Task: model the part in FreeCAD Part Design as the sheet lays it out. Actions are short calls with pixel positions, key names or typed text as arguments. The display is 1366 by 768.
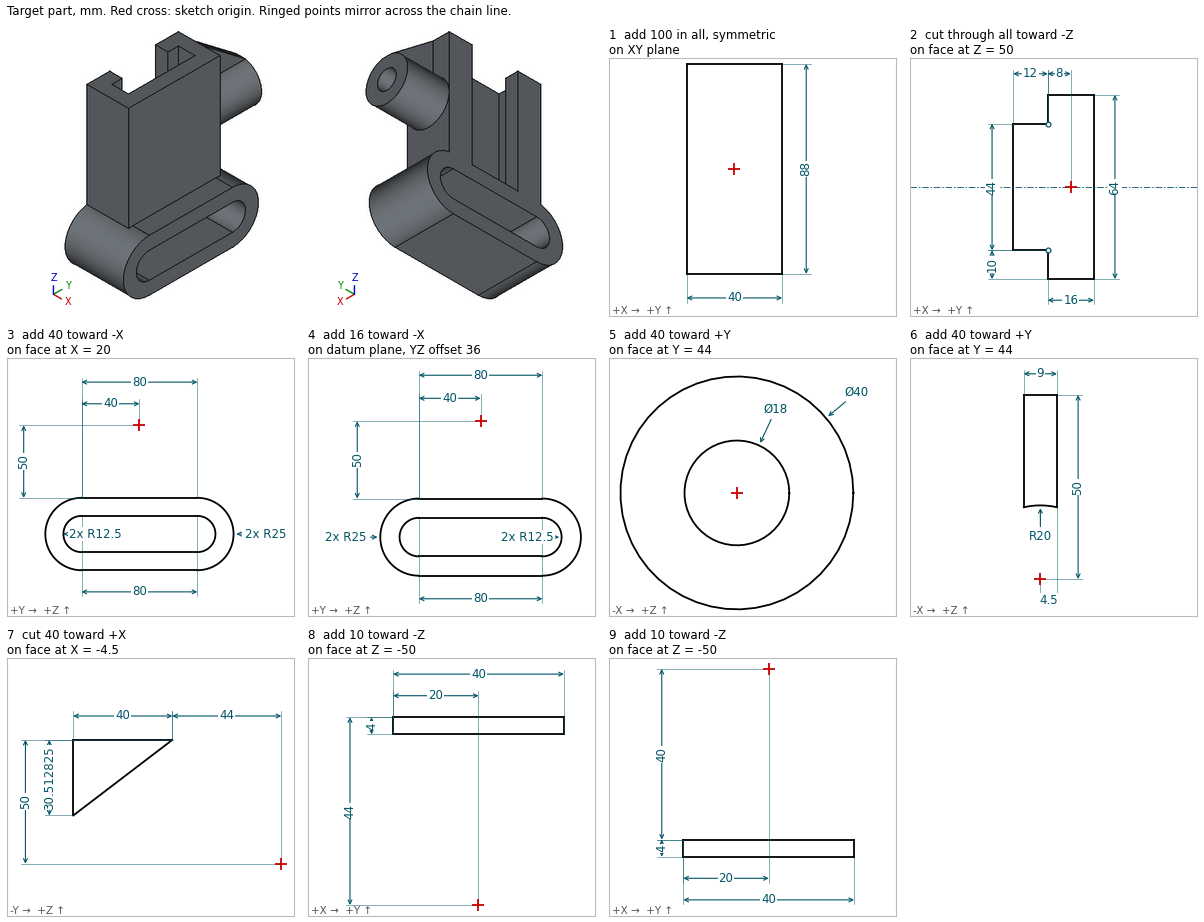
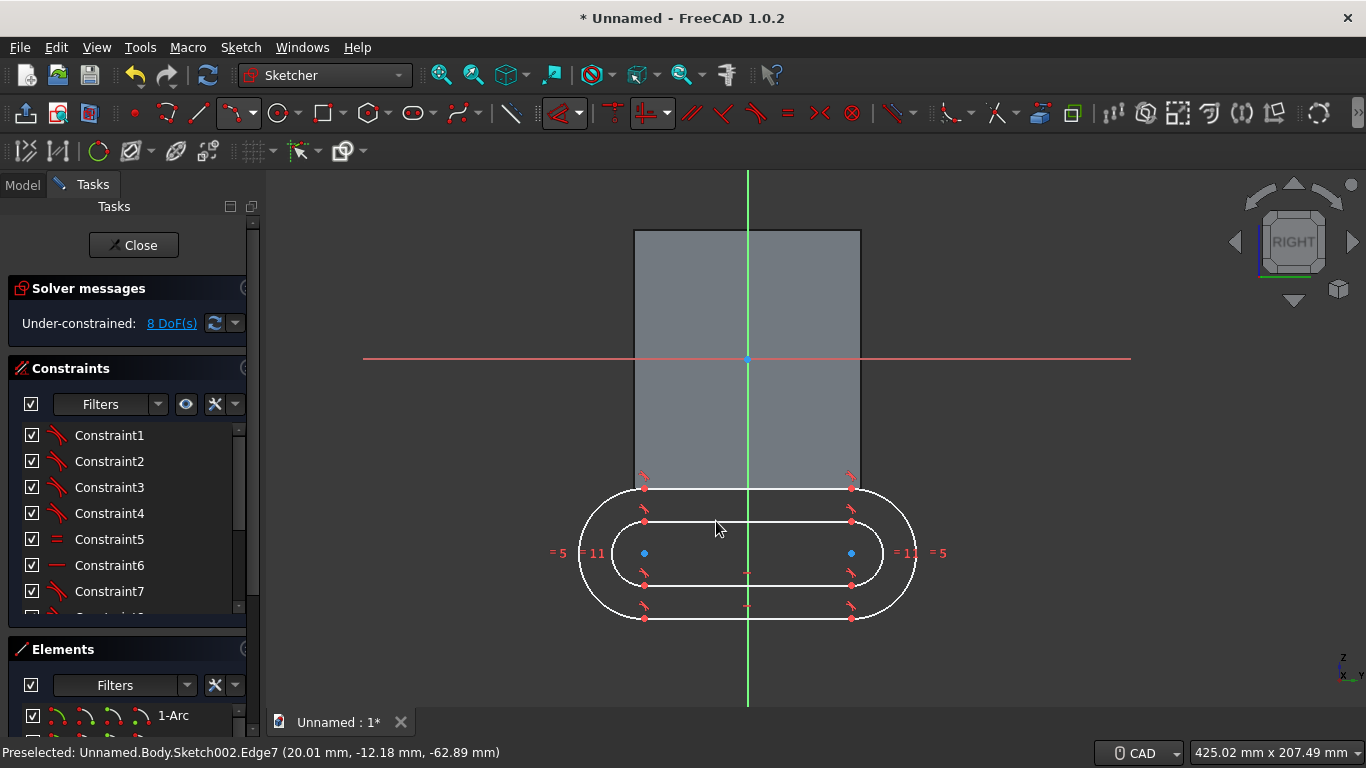
click(591, 516)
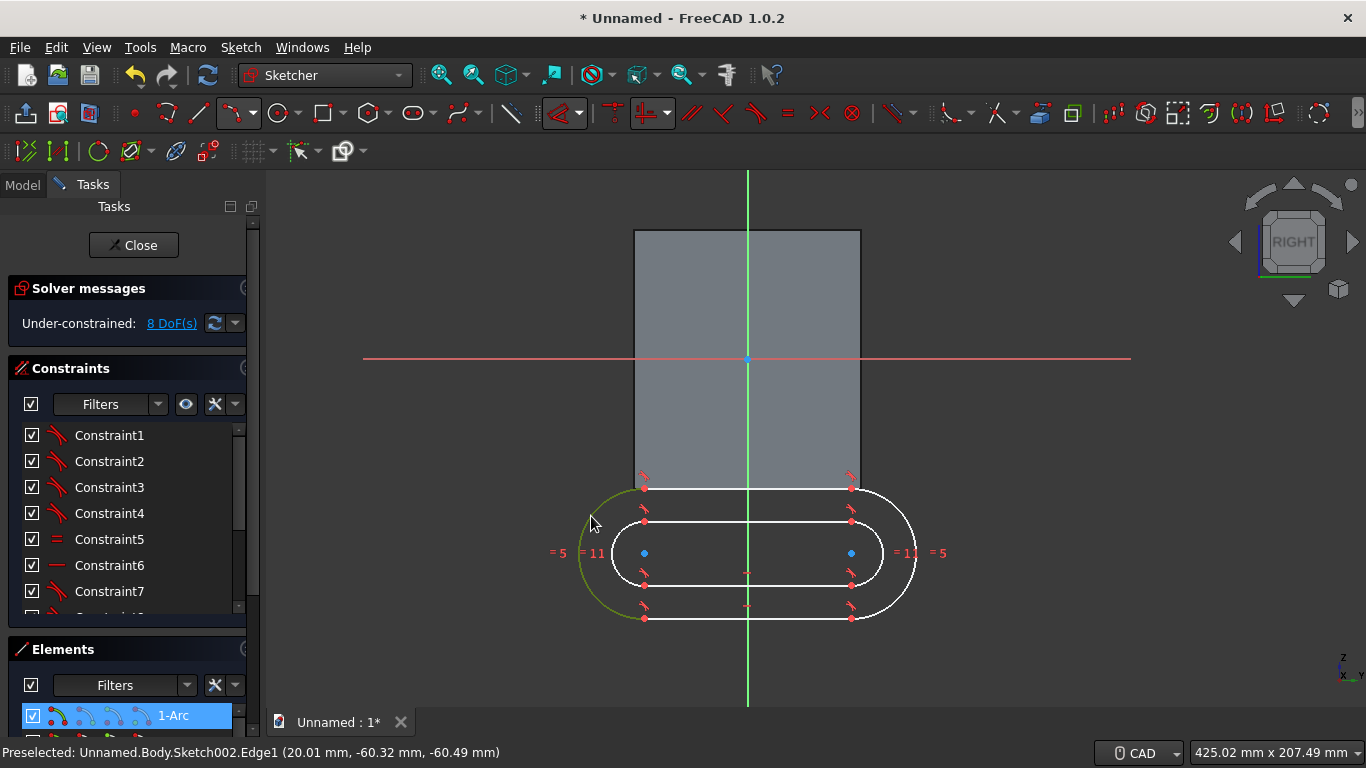
click(618, 535)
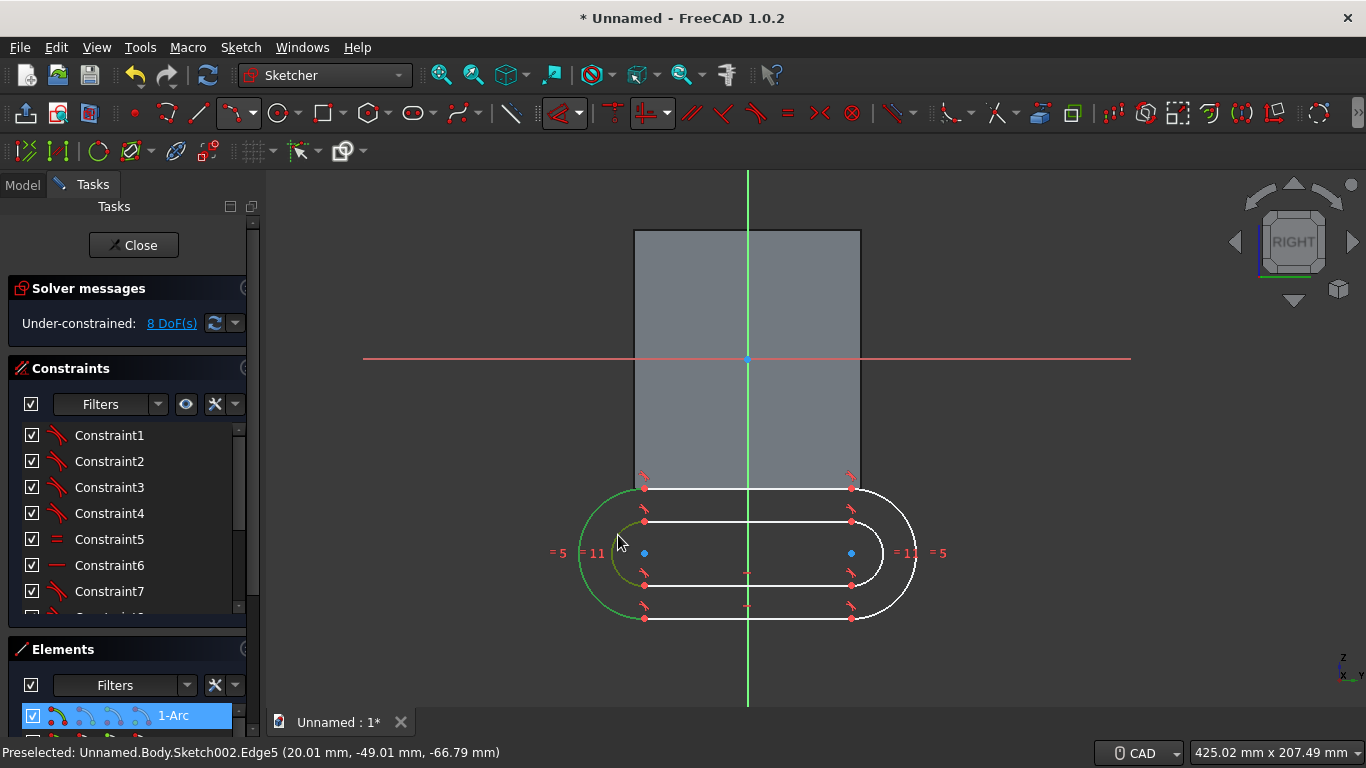
key(c)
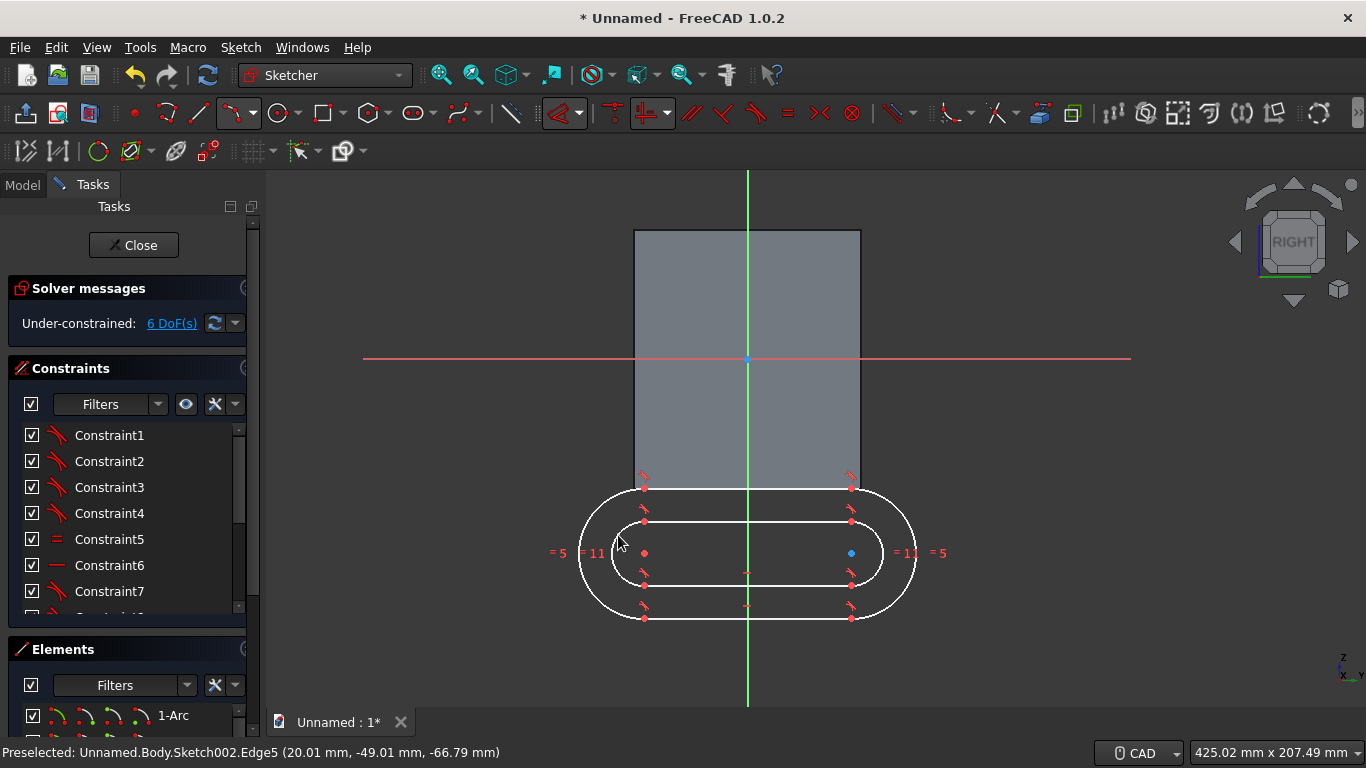
click(591, 516)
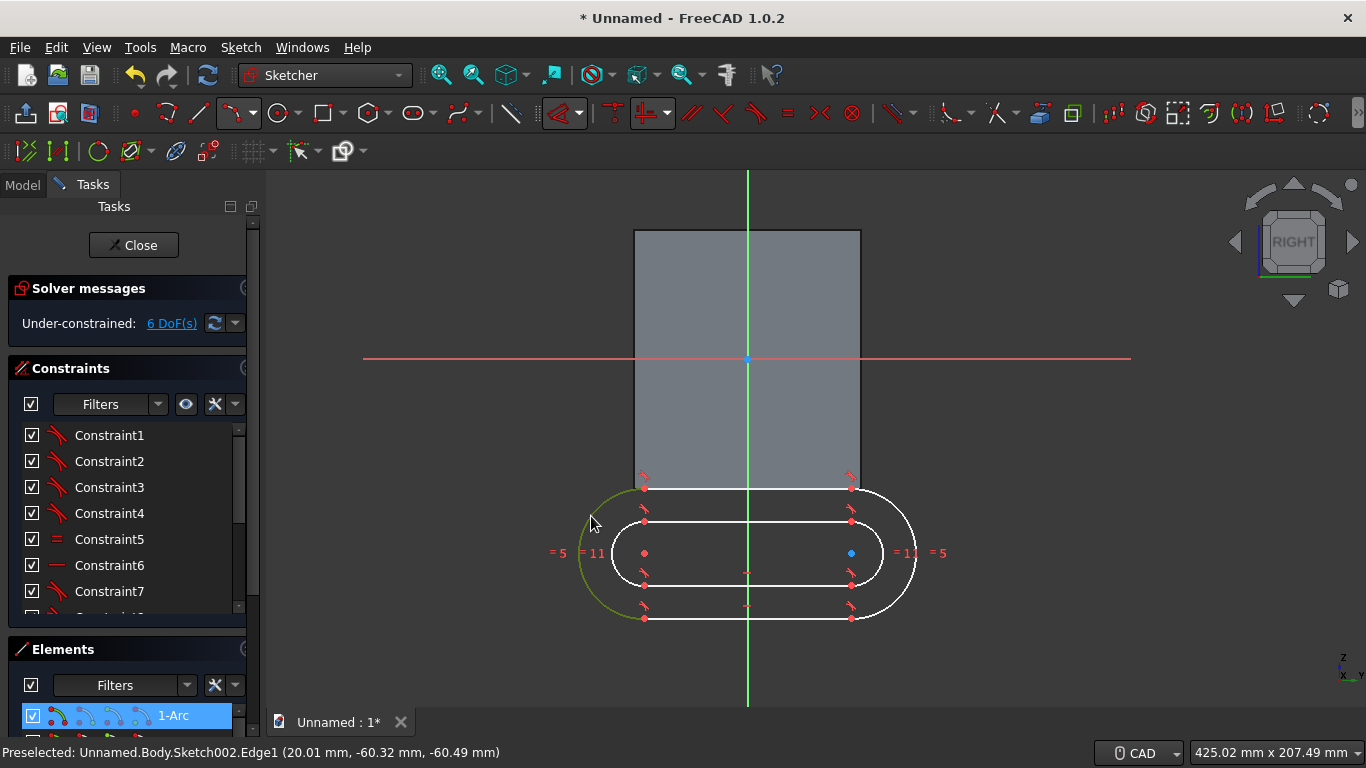
click(582, 114)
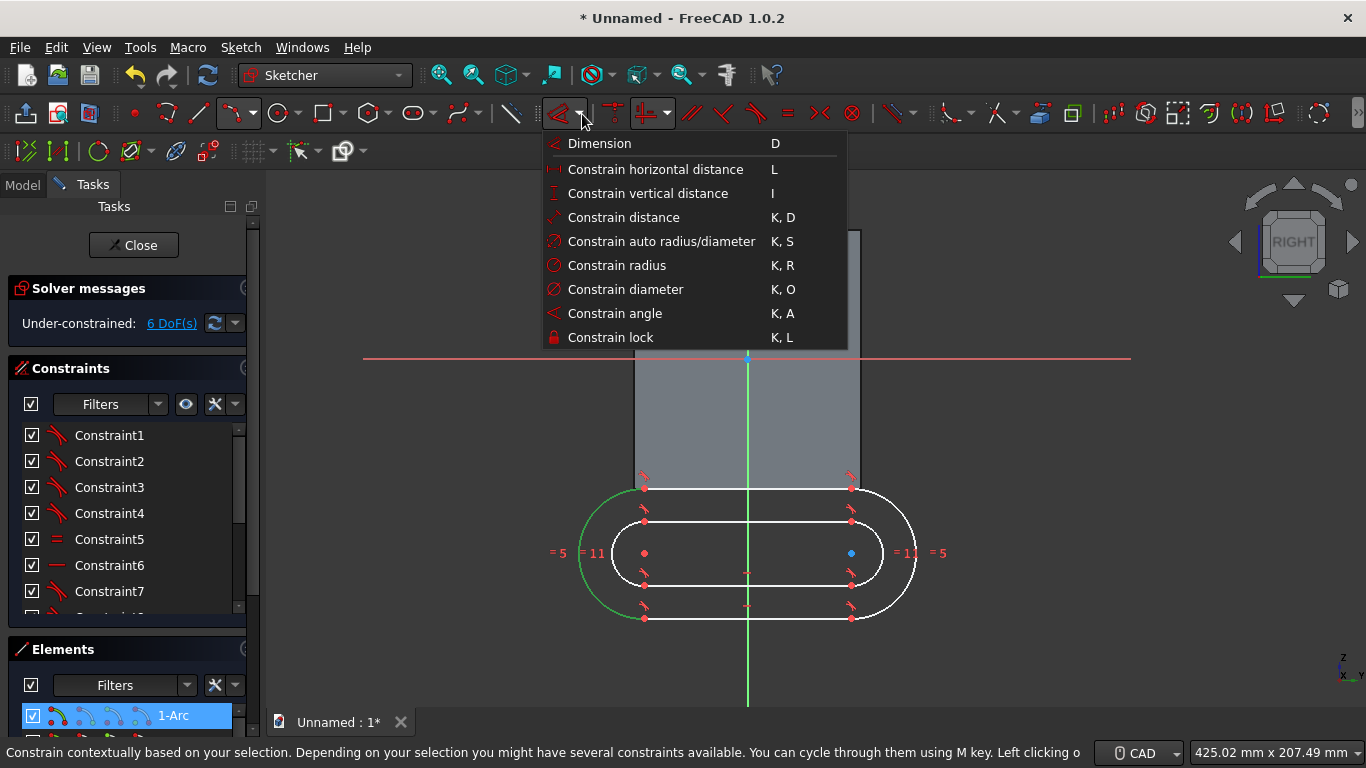
click(695, 265)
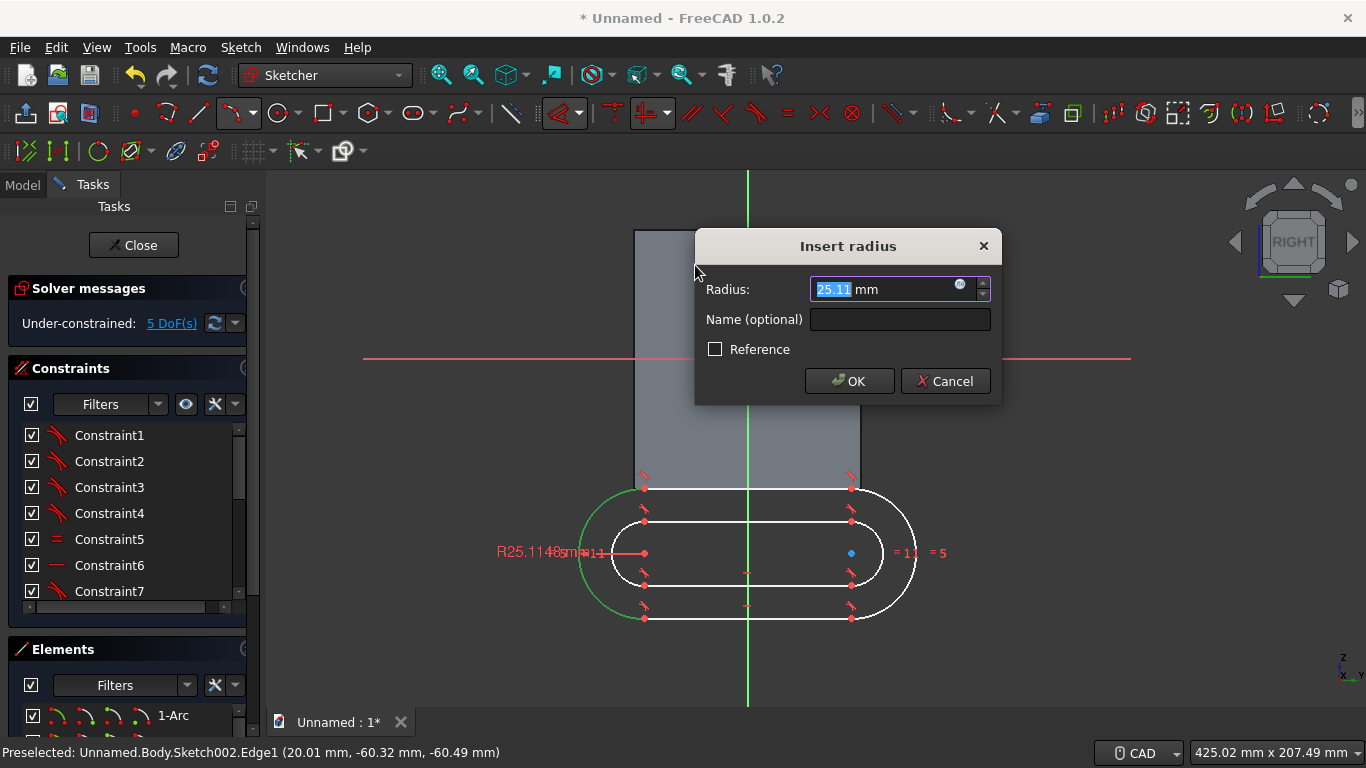
text(25)
key(Return)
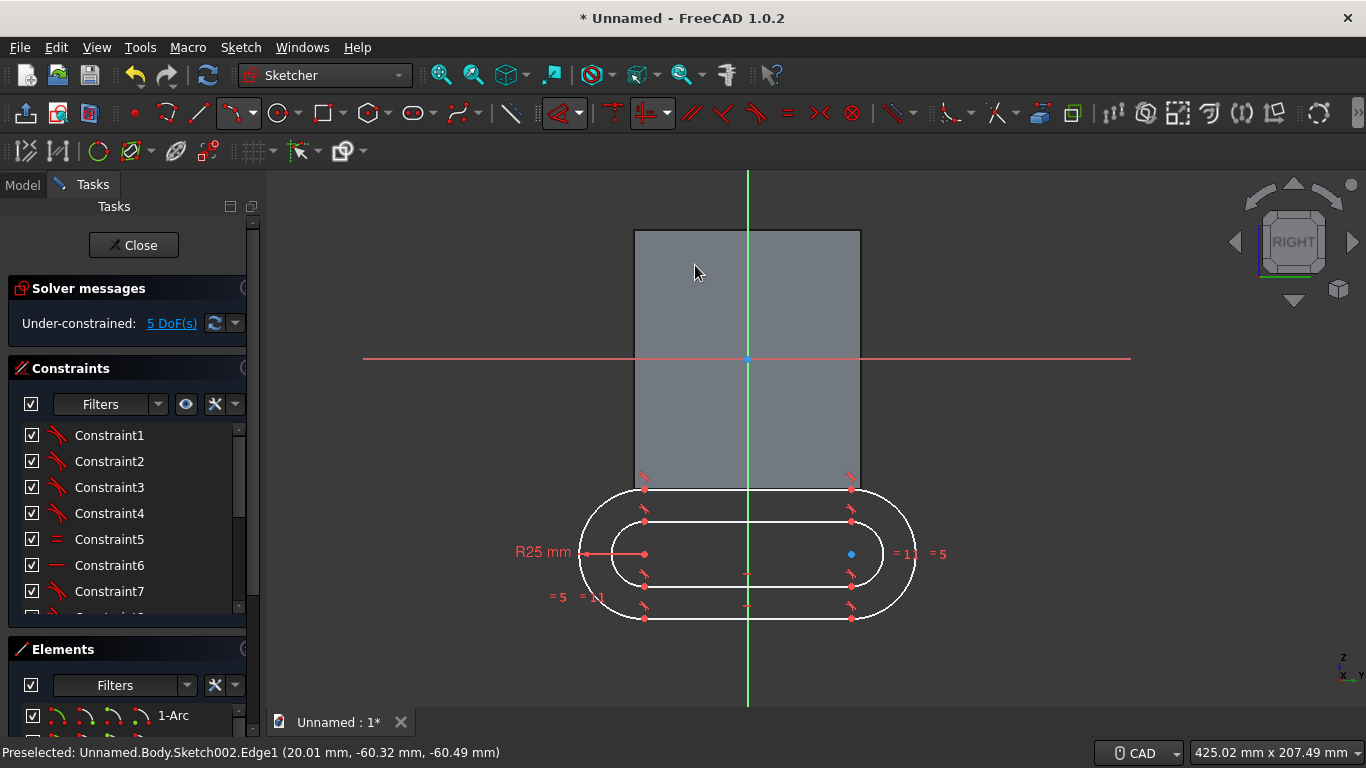
scroll(618, 535, up, 2)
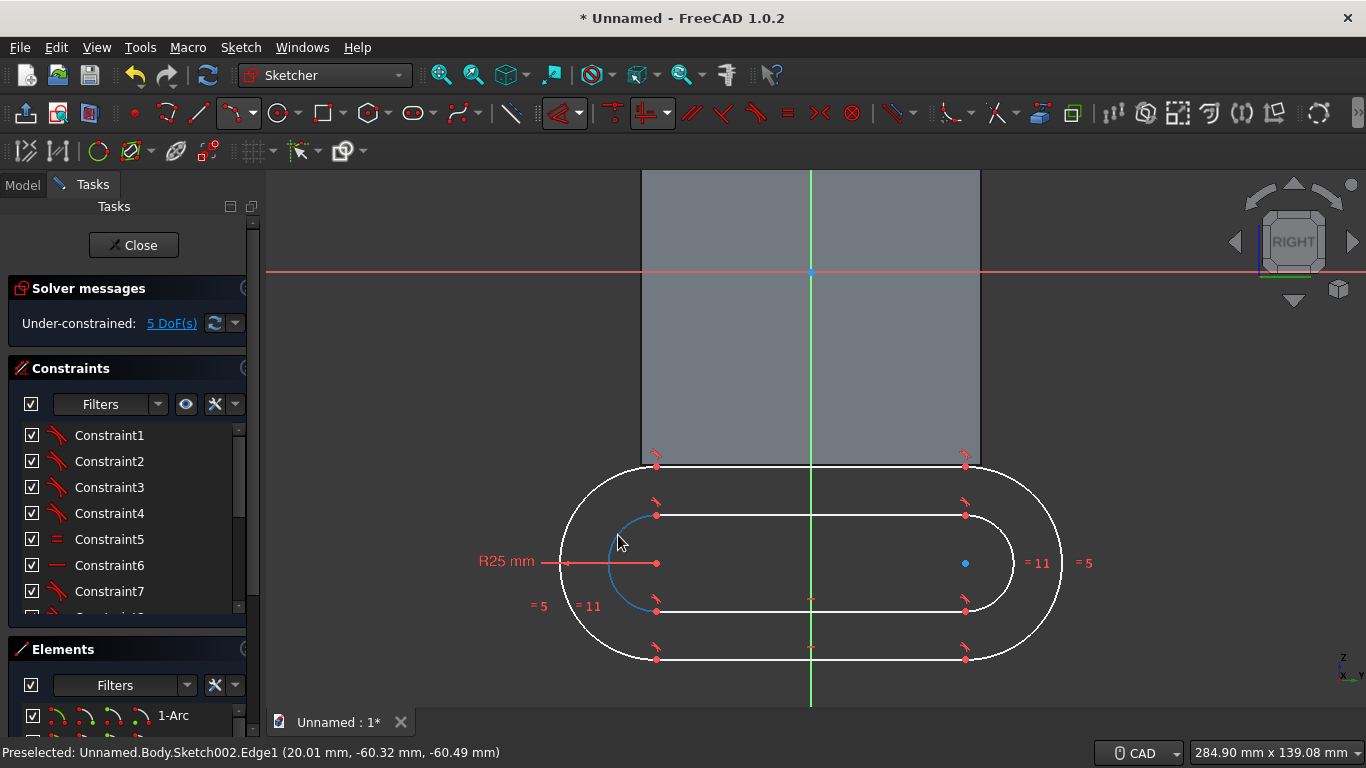
click(618, 535)